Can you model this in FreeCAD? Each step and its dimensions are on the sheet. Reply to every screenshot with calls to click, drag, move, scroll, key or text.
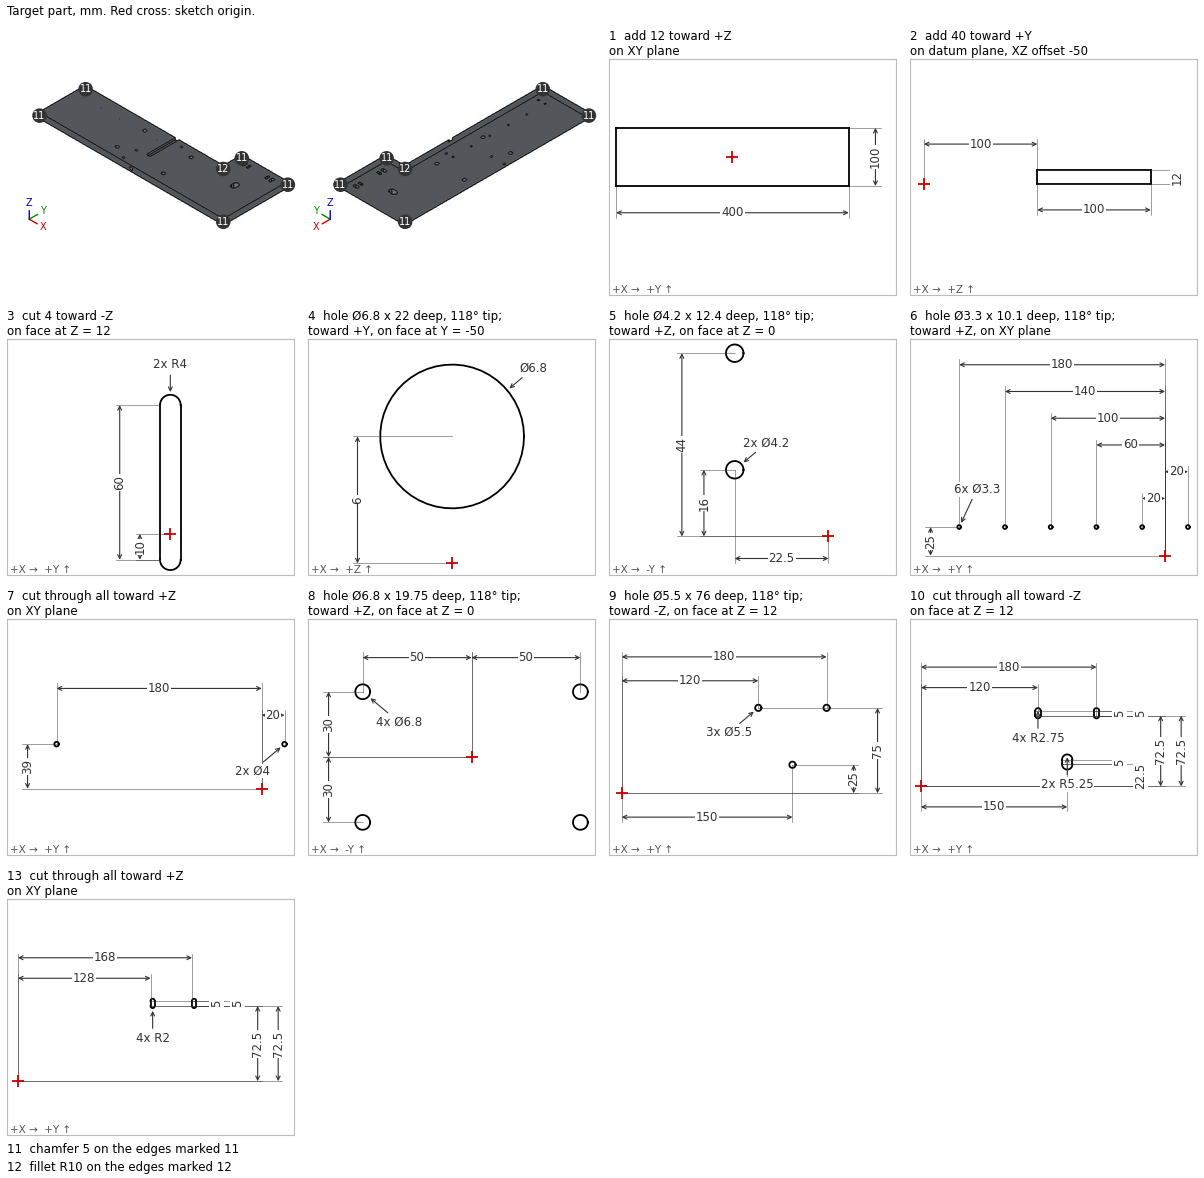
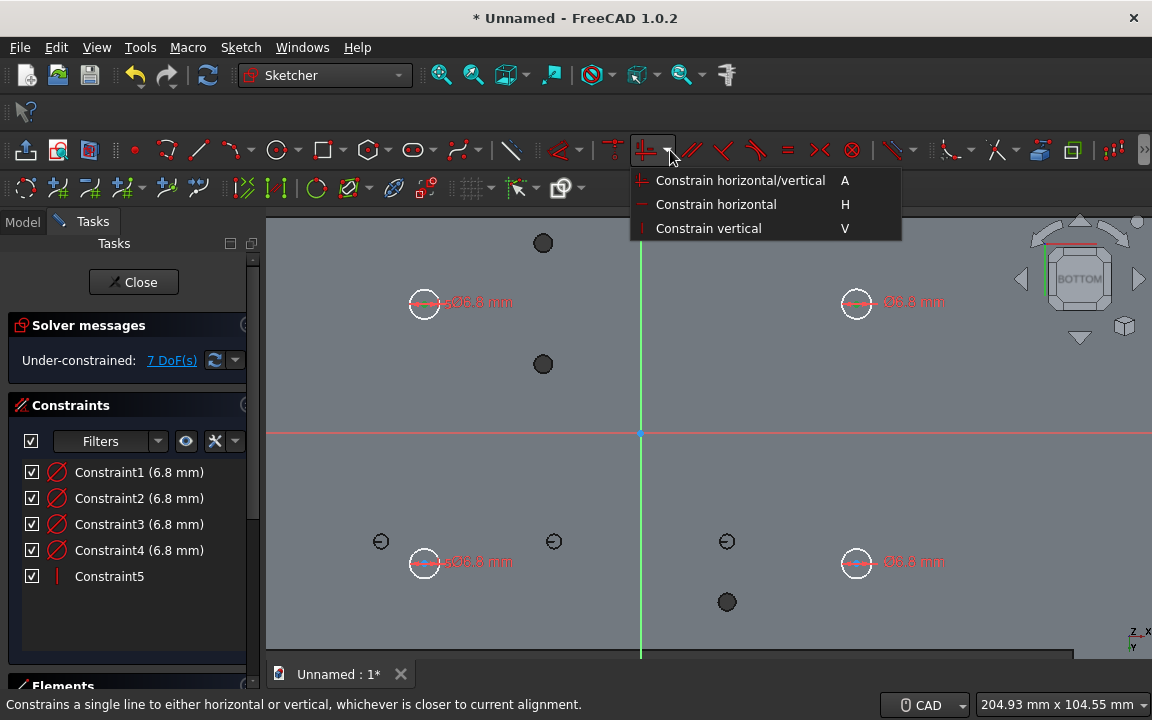
click(766, 204)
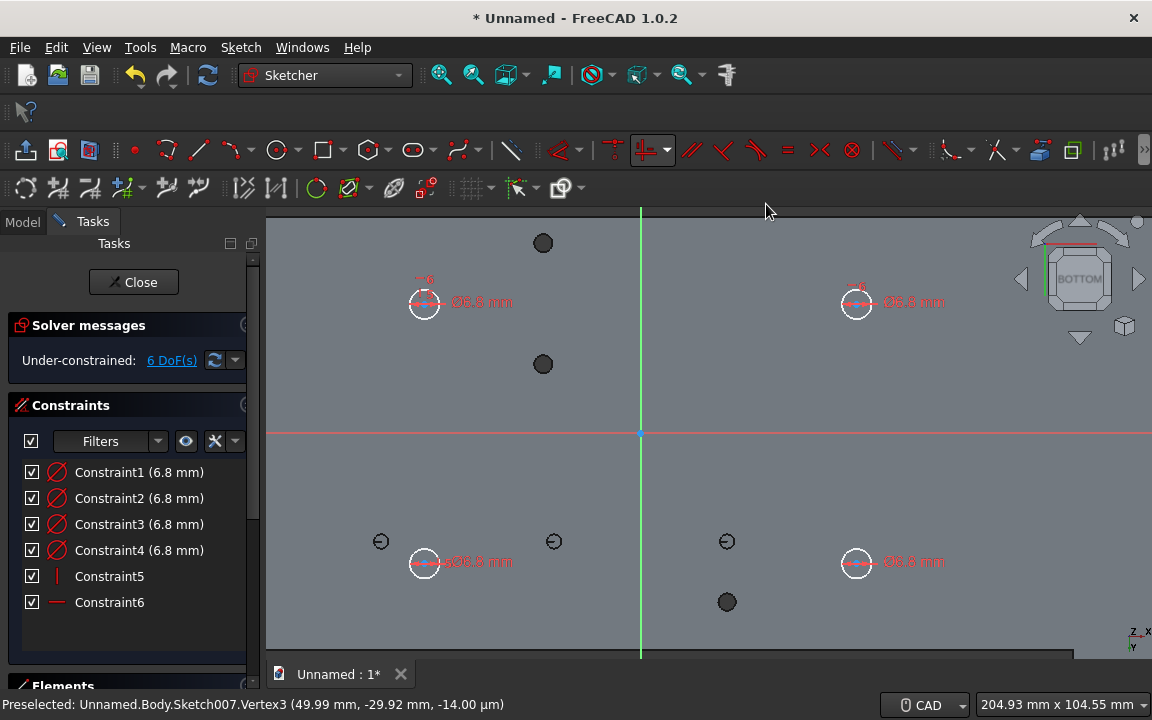
click(857, 304)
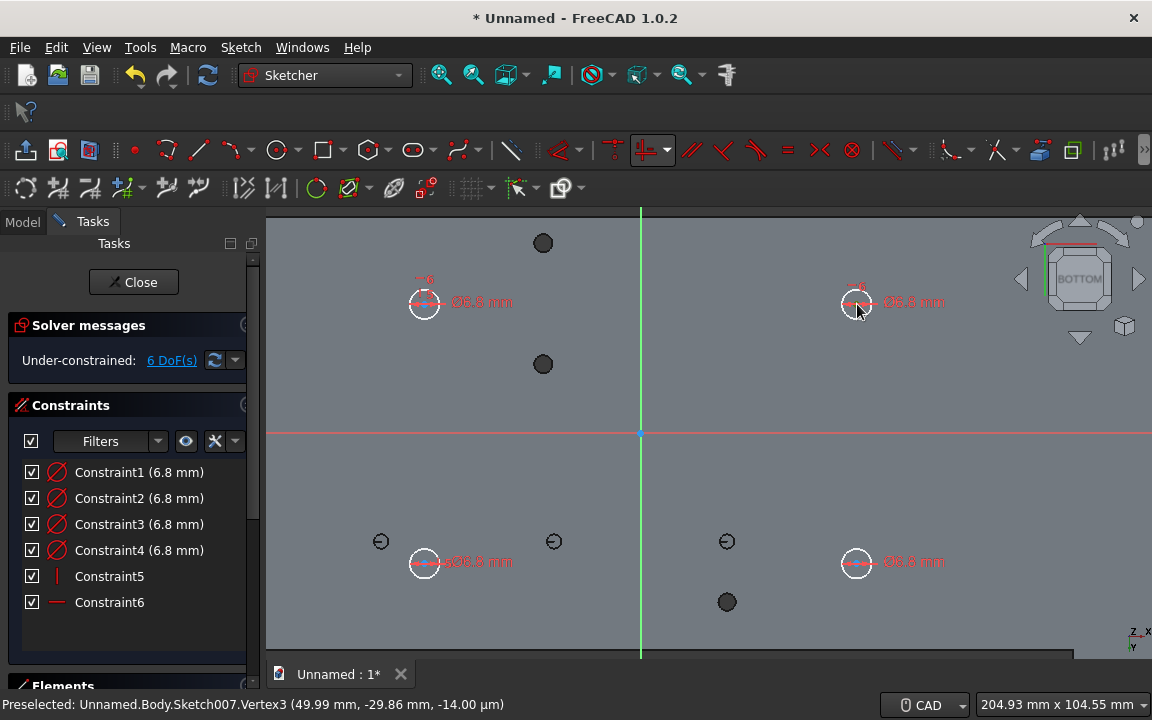
click(857, 564)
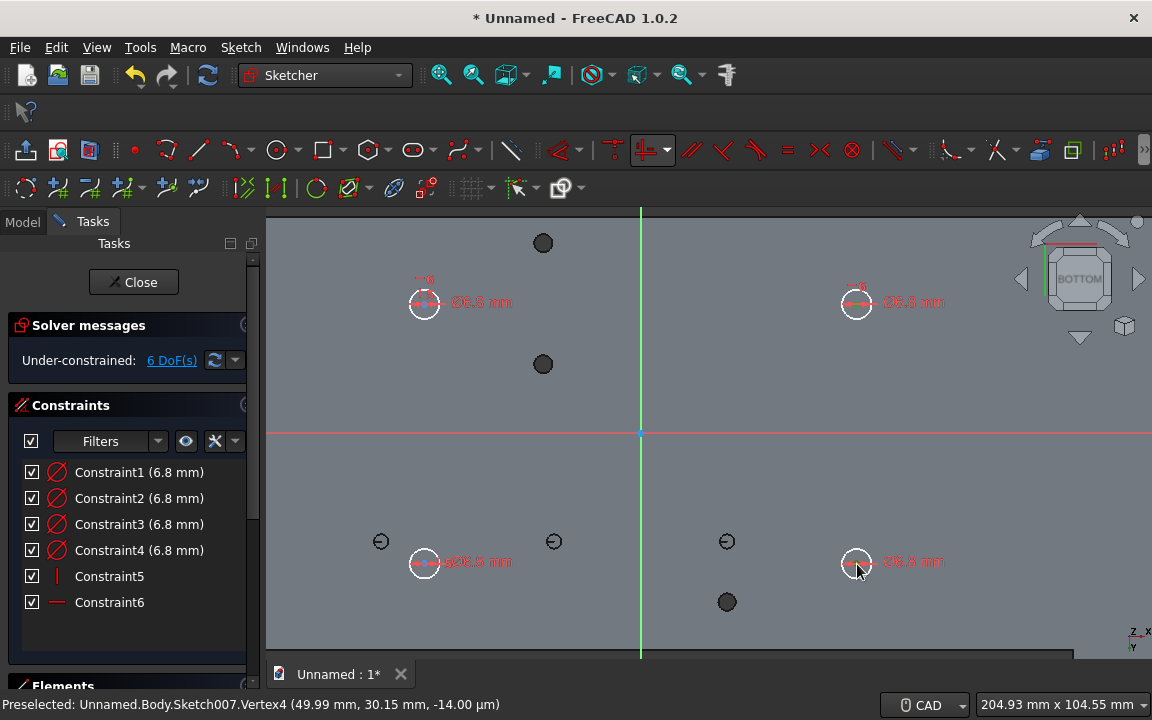
key(v)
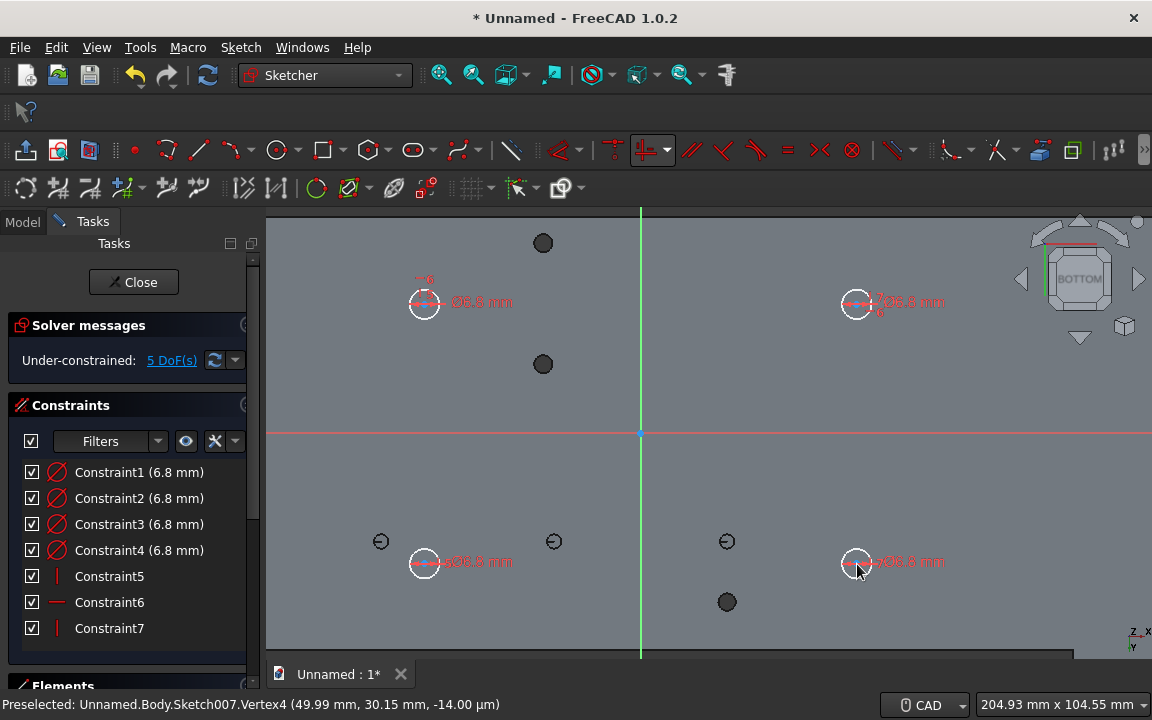
click(425, 564)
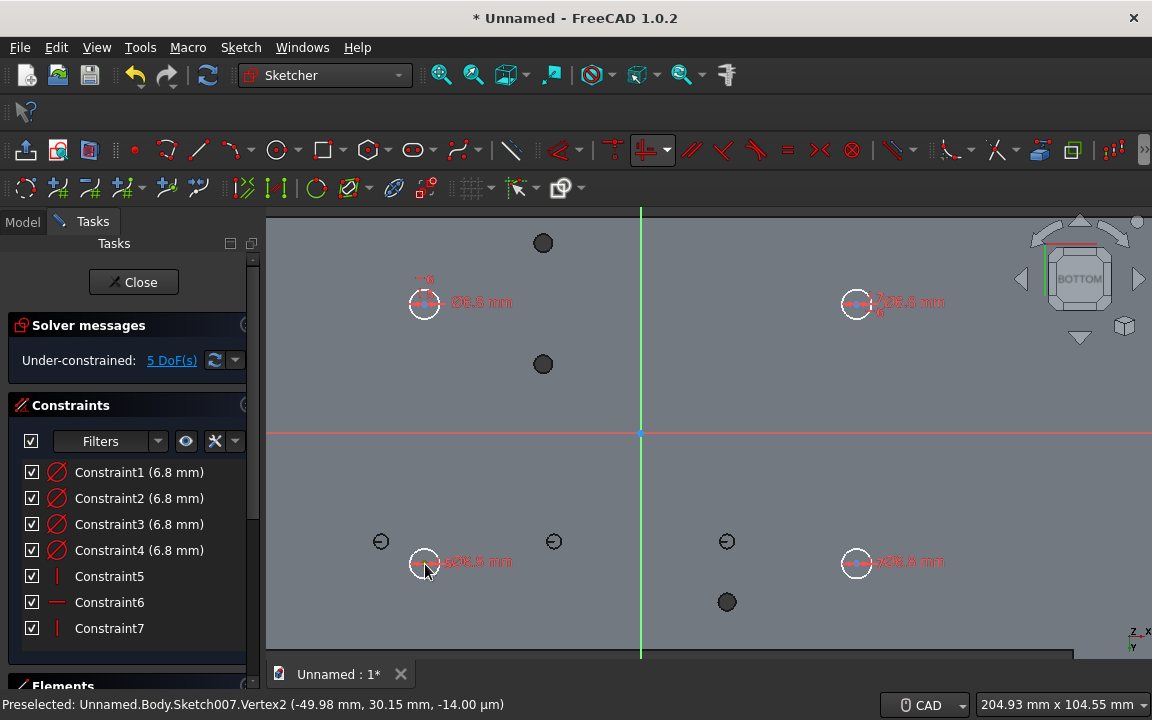
click(857, 564)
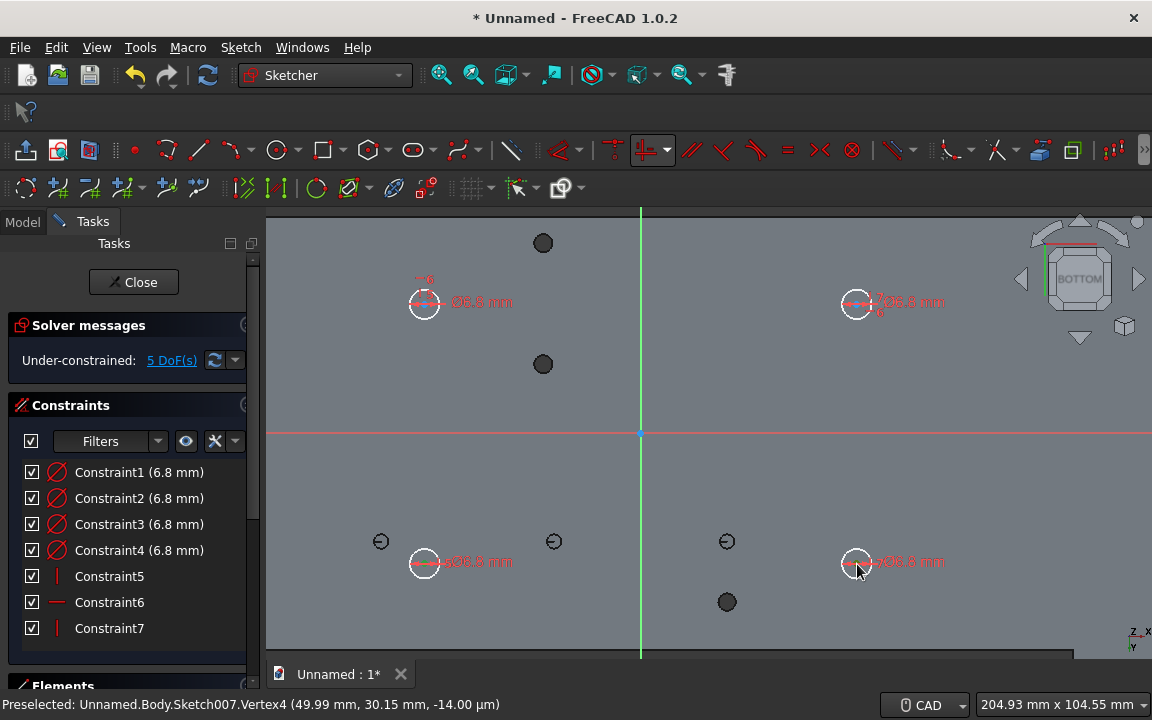
click(670, 150)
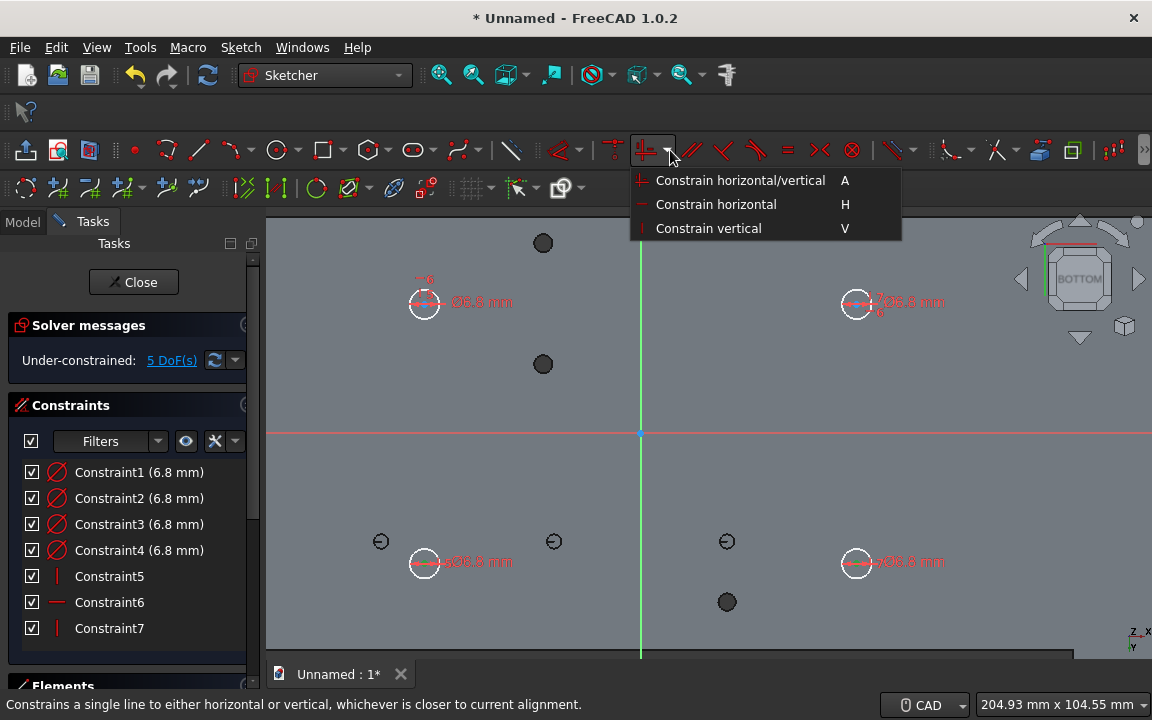
click(766, 204)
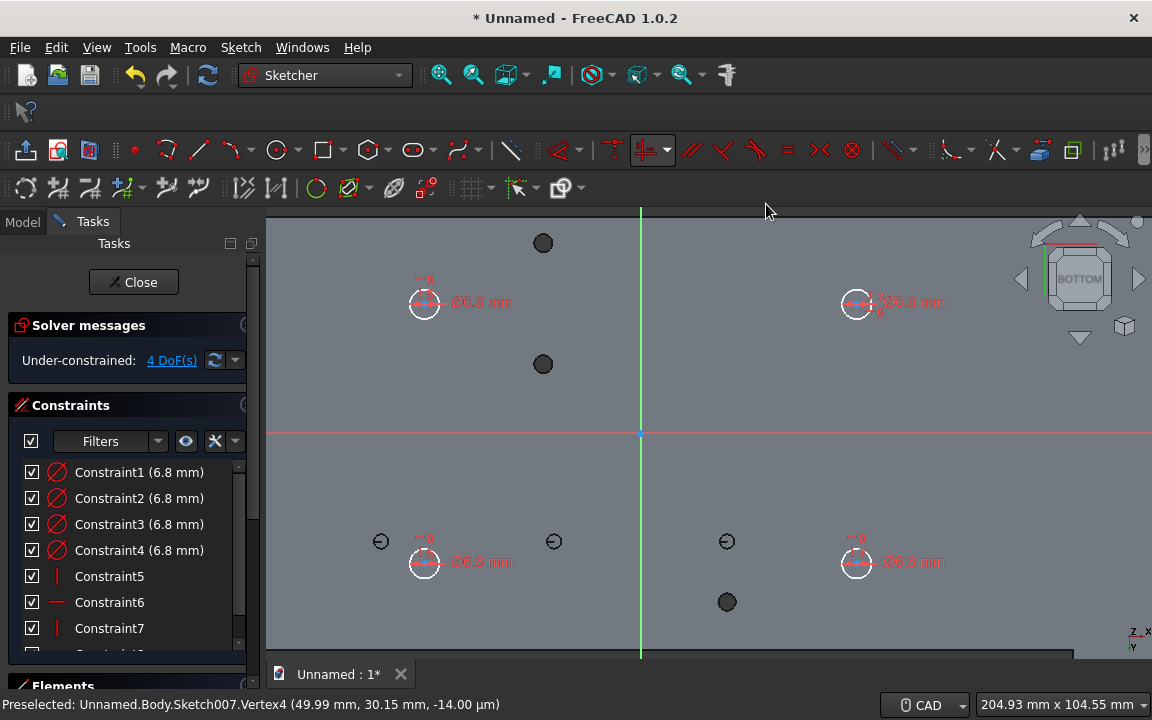
click(558, 150)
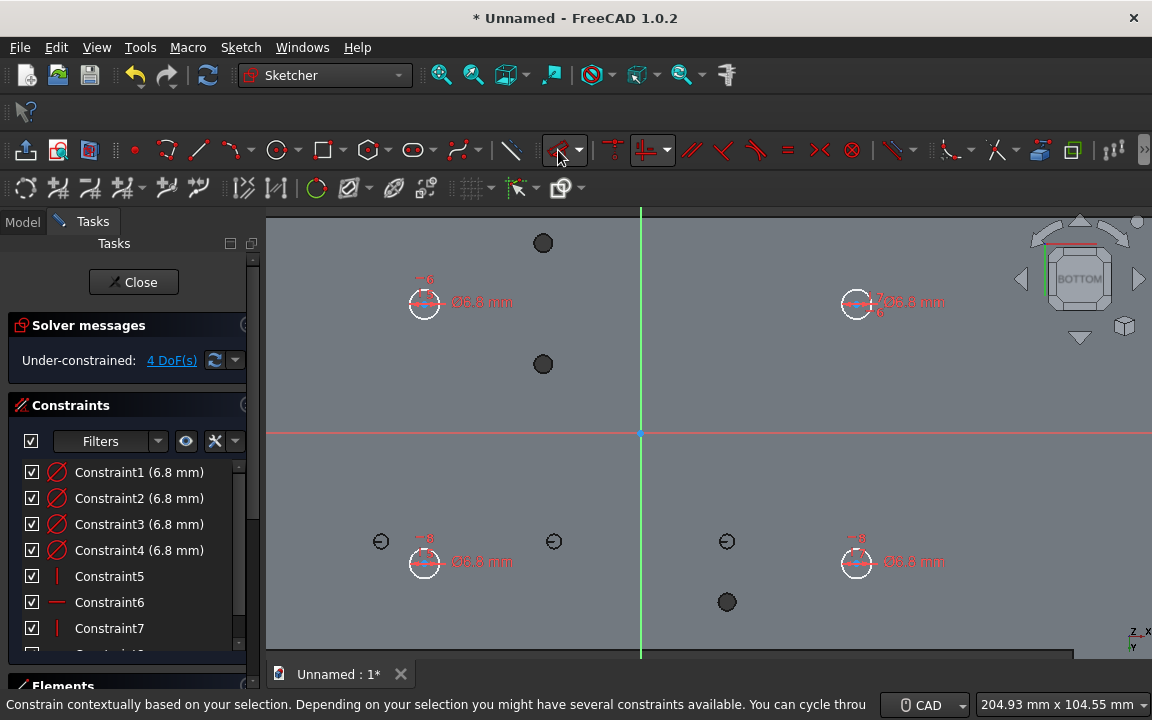
click(425, 304)
click(533, 270)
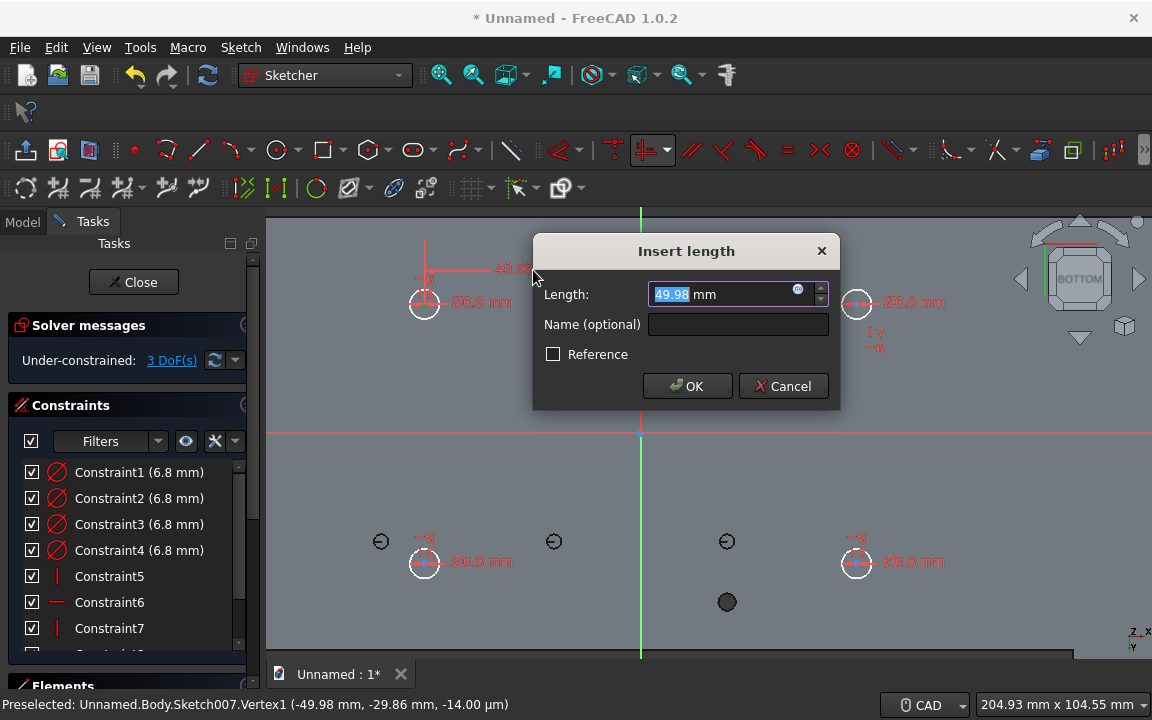
text(50)
key(Return)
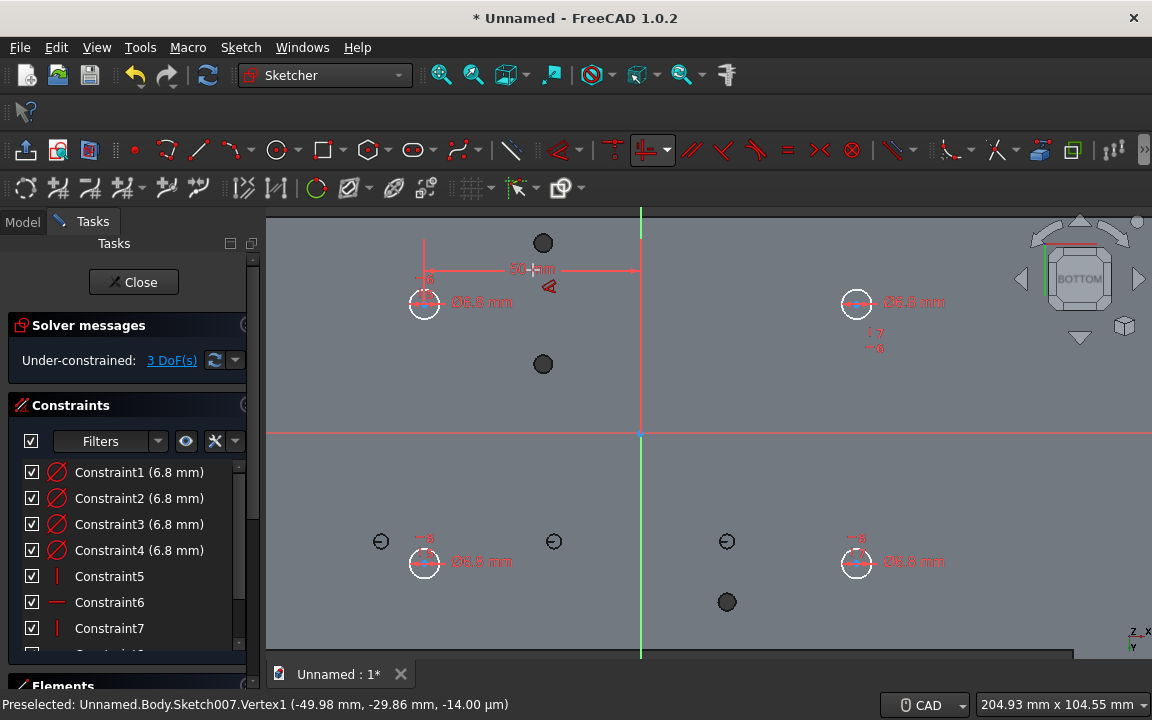
click(424, 304)
click(390, 369)